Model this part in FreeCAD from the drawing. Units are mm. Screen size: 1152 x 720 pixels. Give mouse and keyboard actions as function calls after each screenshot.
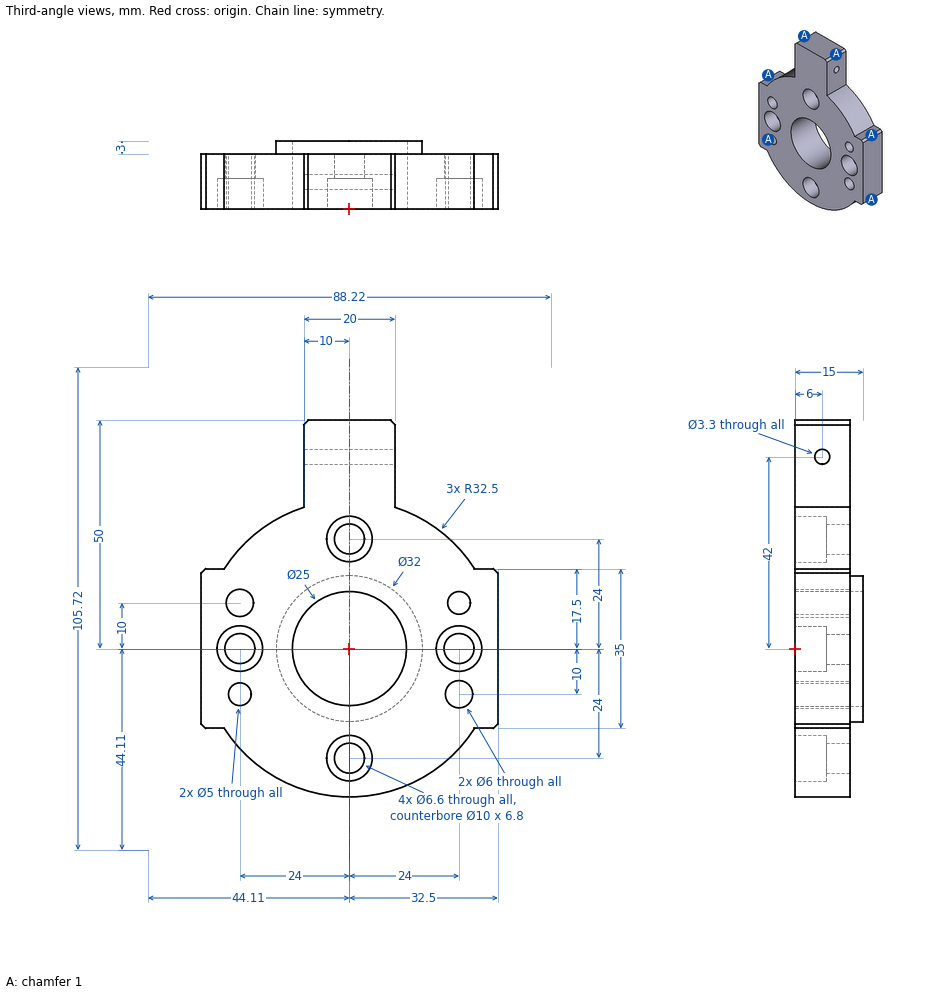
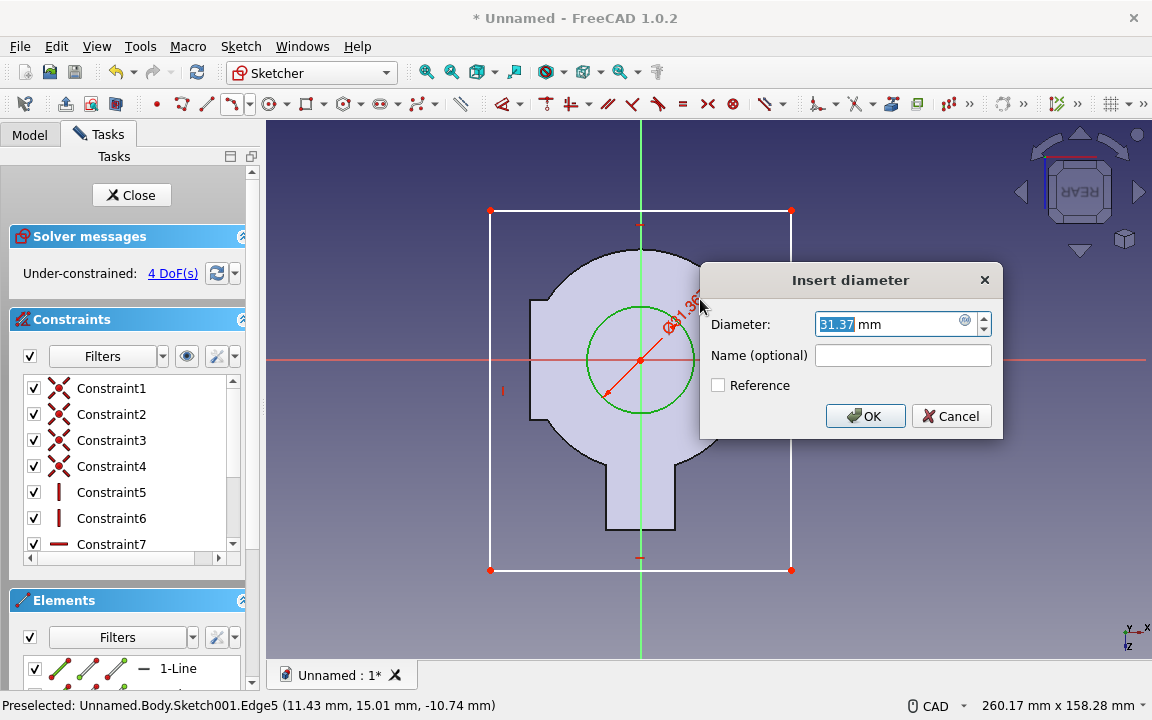
text(32)
key(Return)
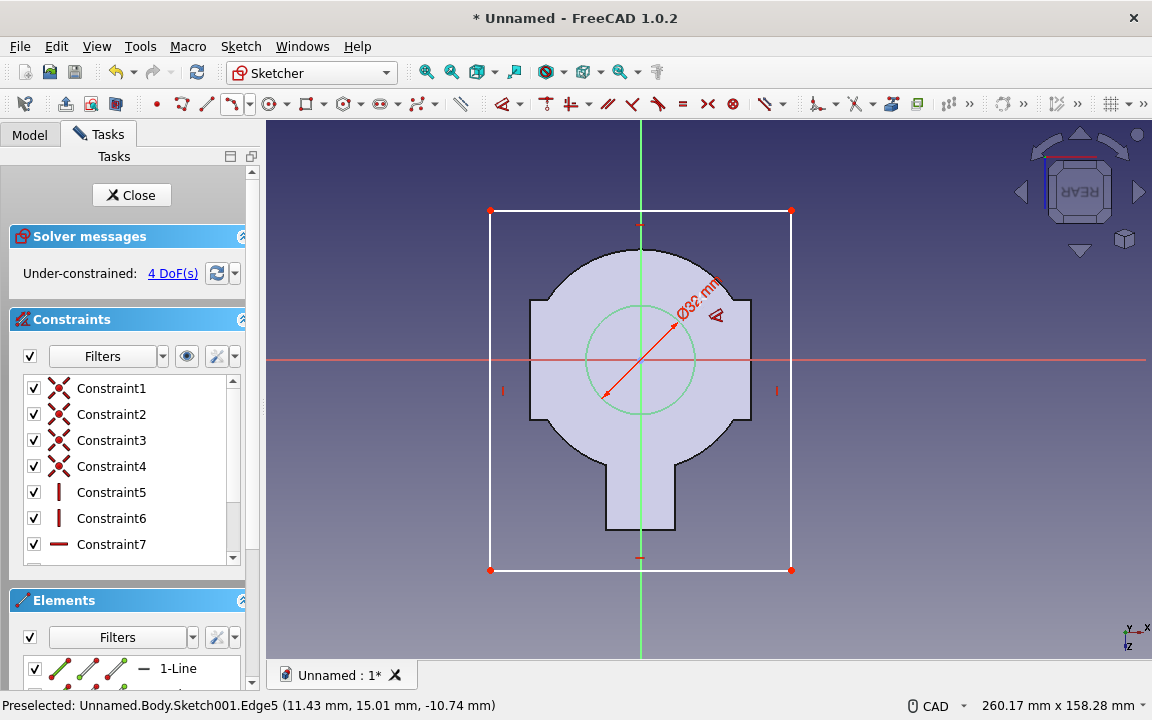
click(580, 571)
click(571, 605)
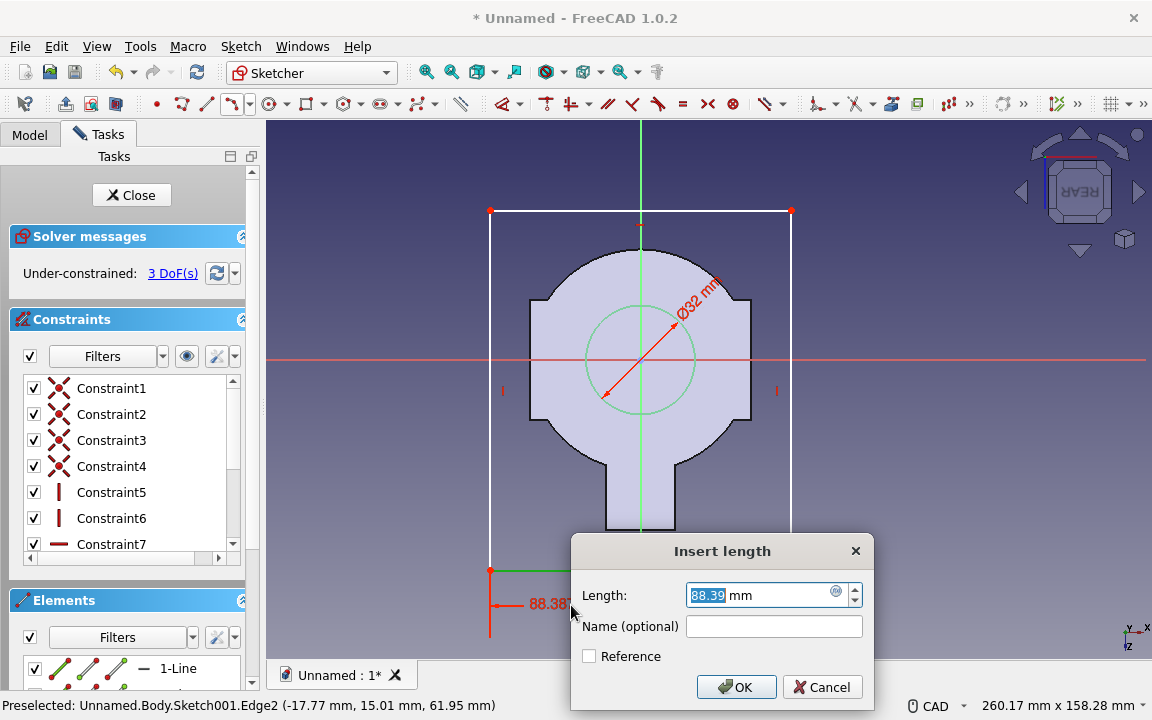
text(88.22)
key(Return)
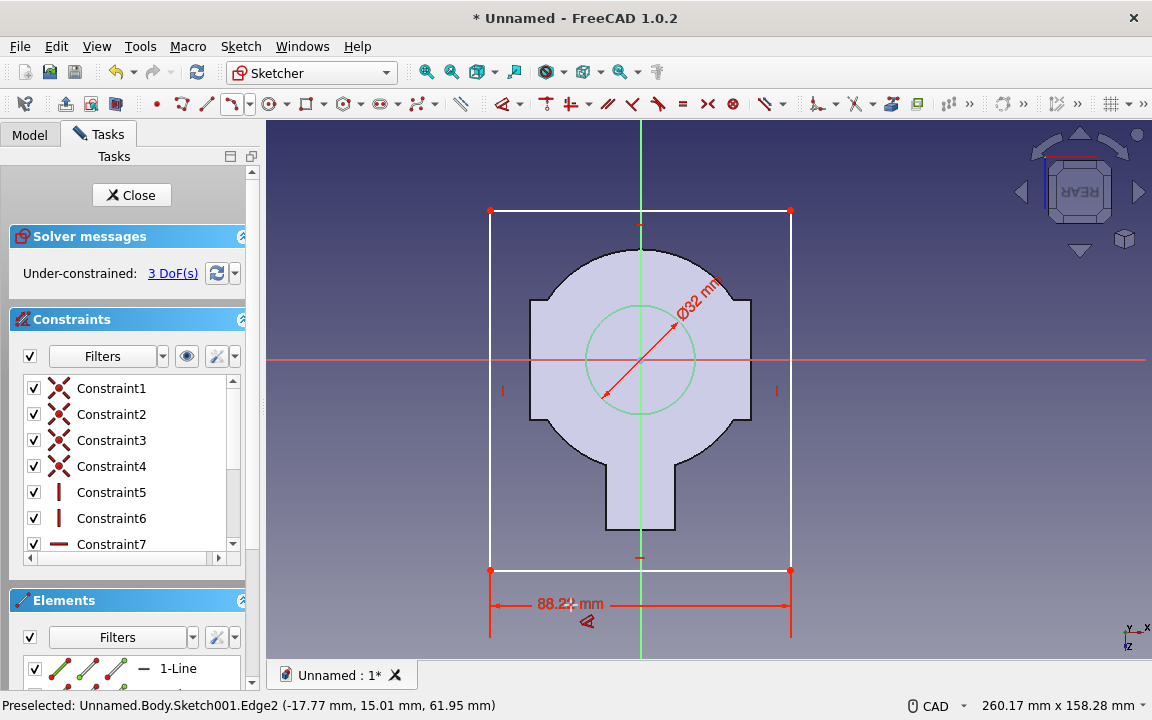
click(490, 319)
click(456, 391)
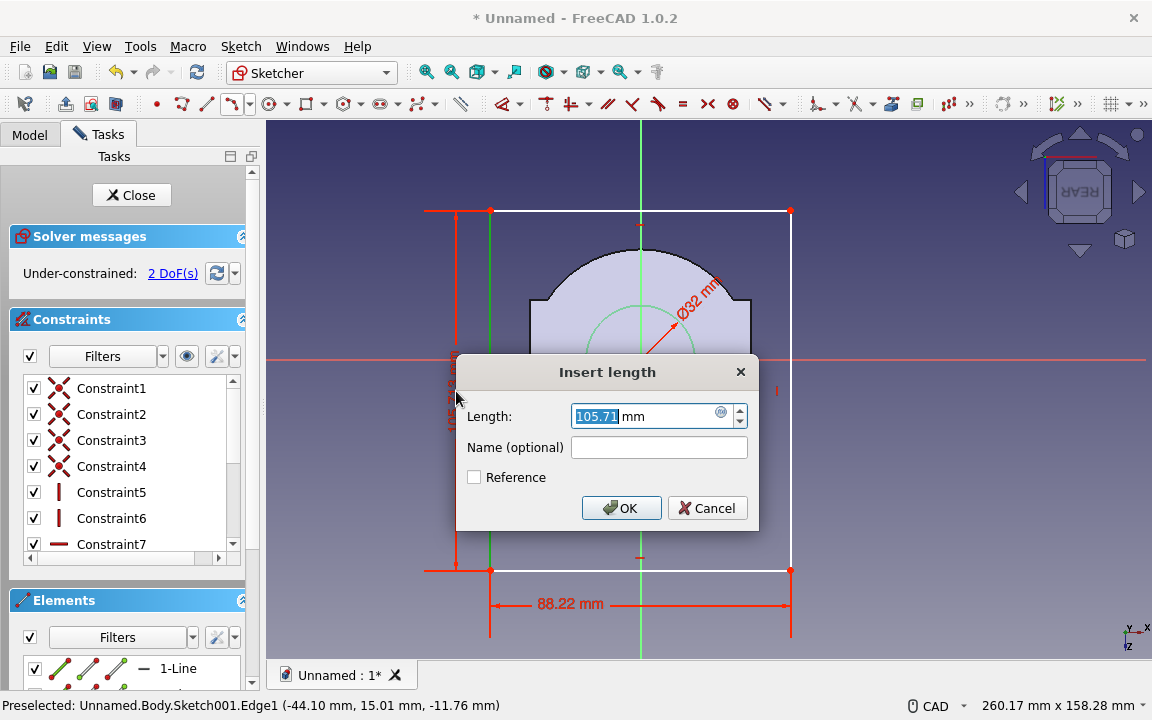
text(105.72)
key(Return)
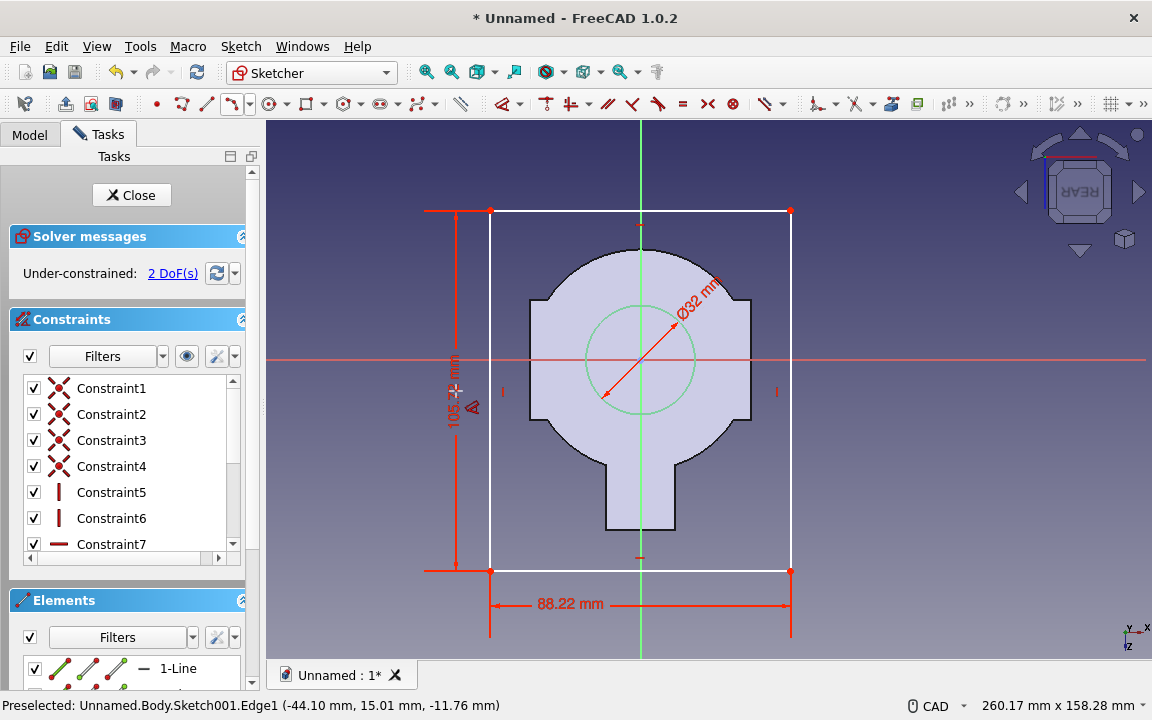
click(490, 211)
click(565, 177)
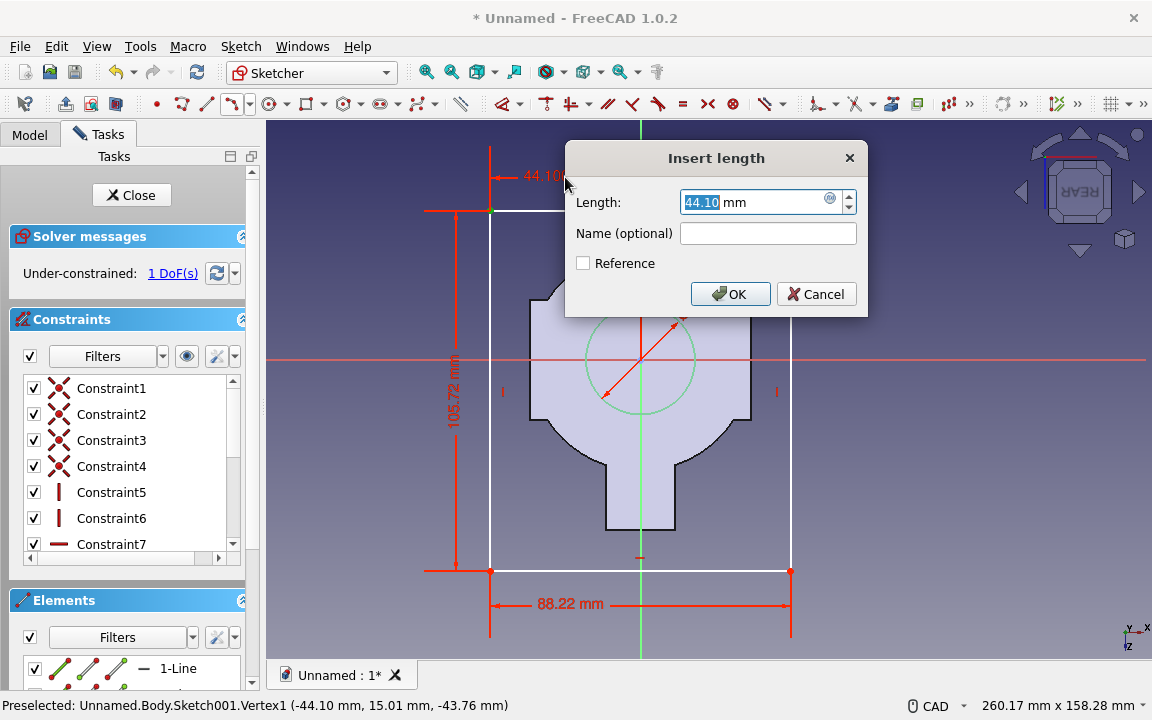
text(44.11)
key(Return)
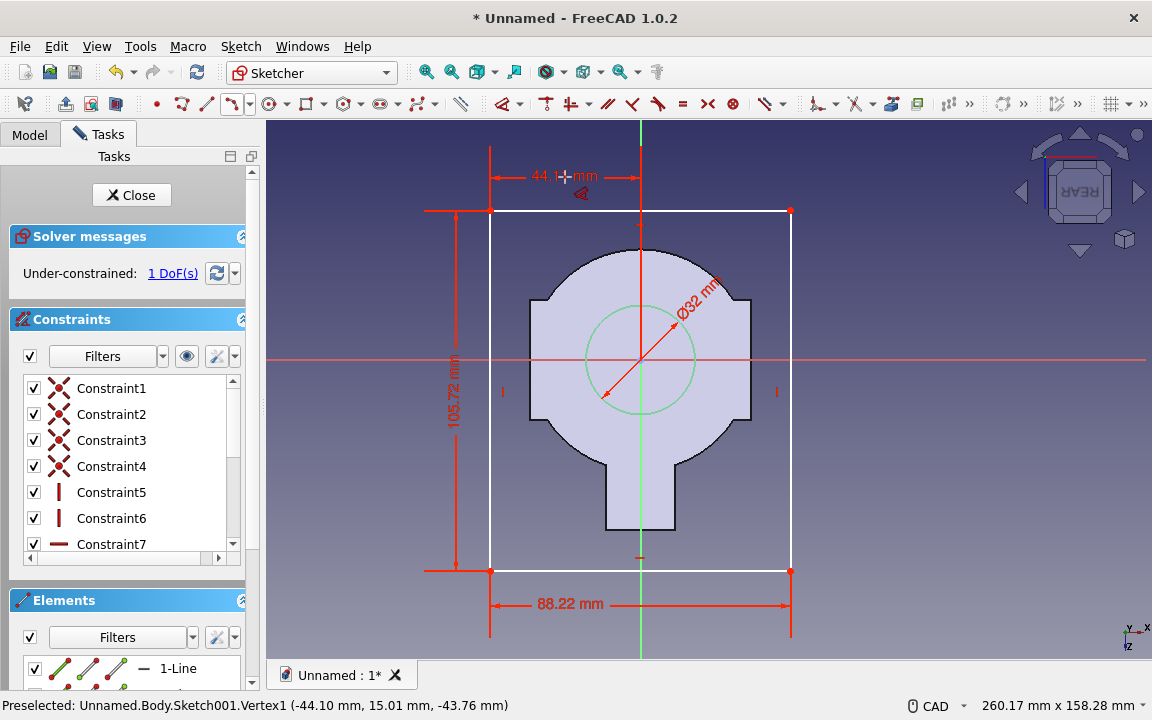
click(490, 211)
click(456, 286)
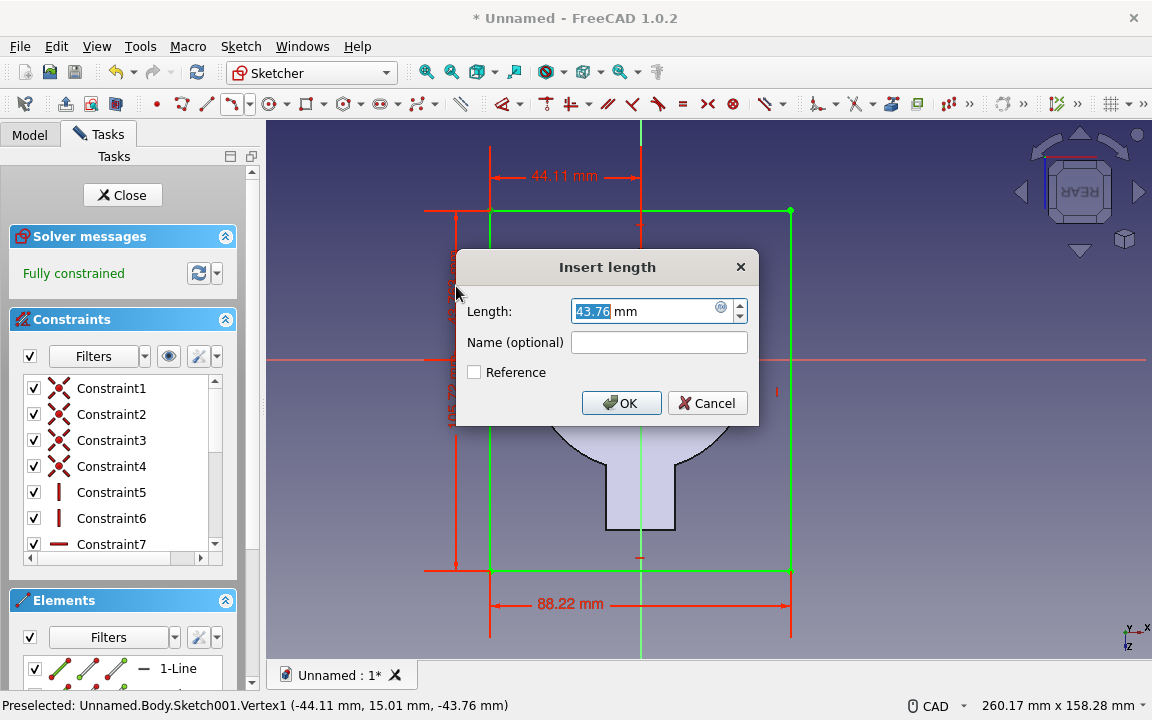
text(44.11)
key(Return)
key(Escape)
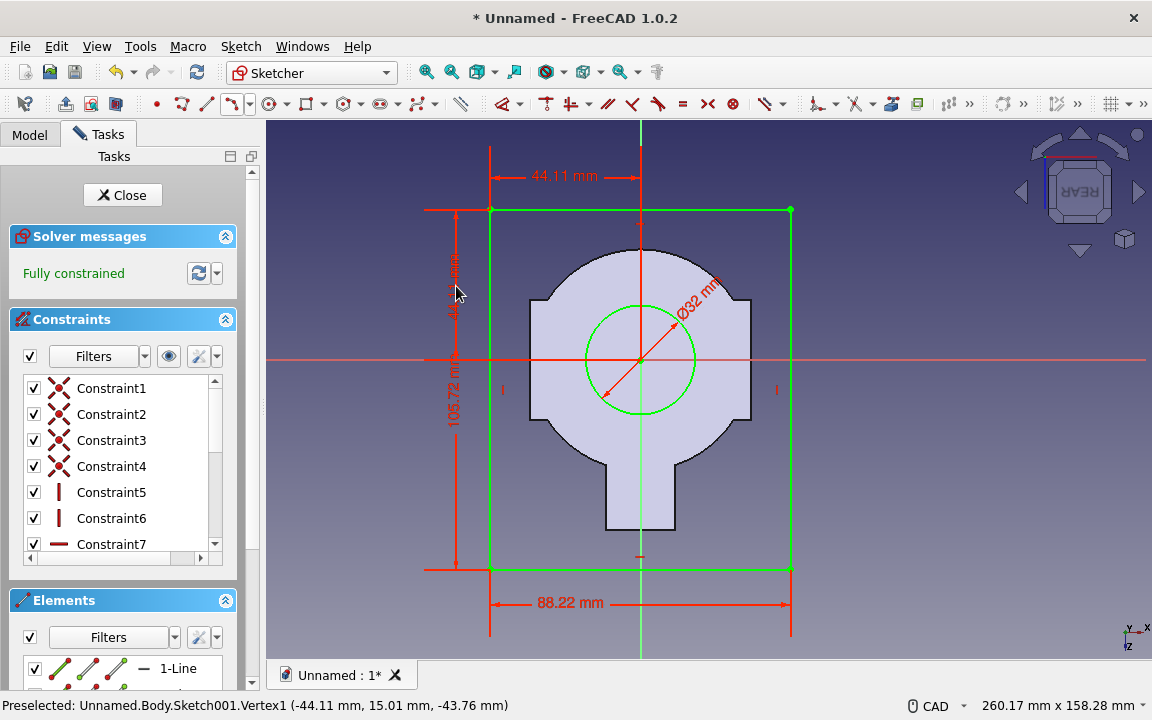
click(123, 195)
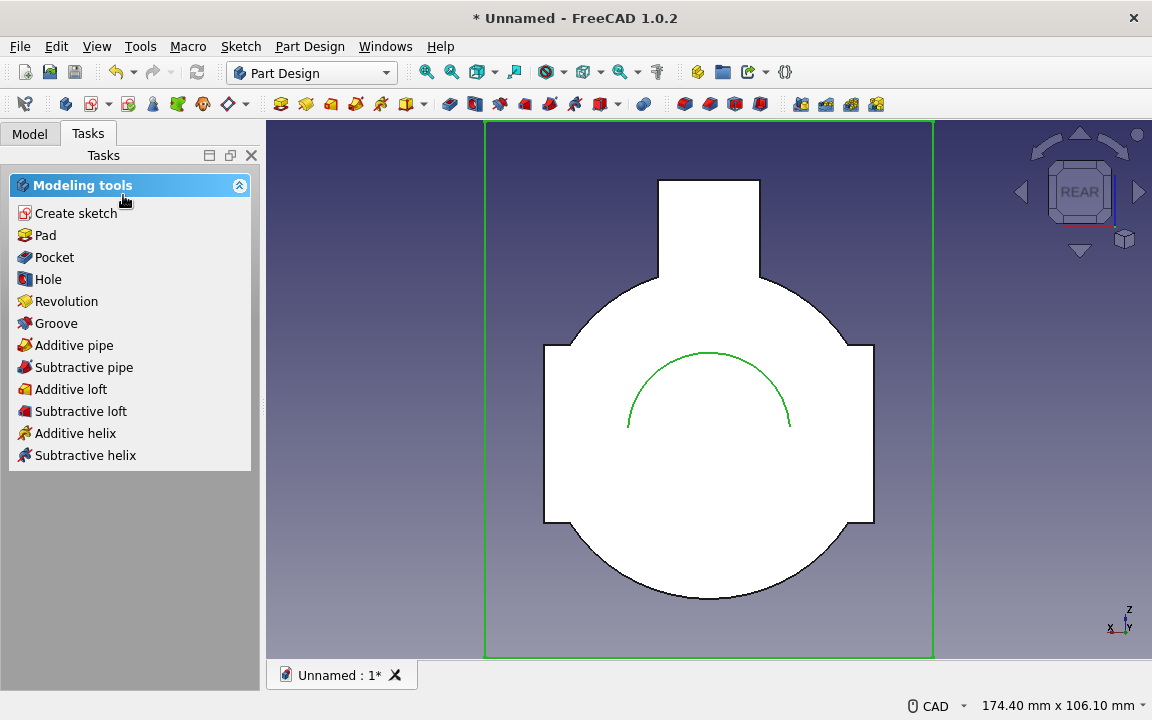
click(450, 104)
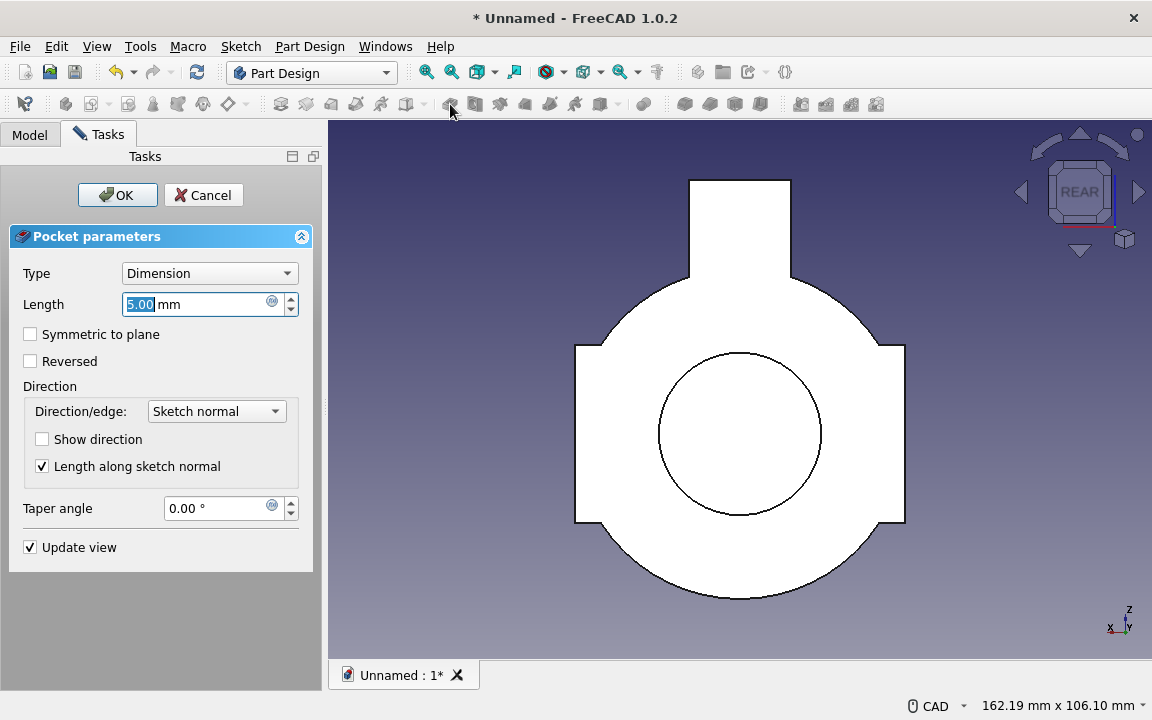
text(3)
key(Tab)